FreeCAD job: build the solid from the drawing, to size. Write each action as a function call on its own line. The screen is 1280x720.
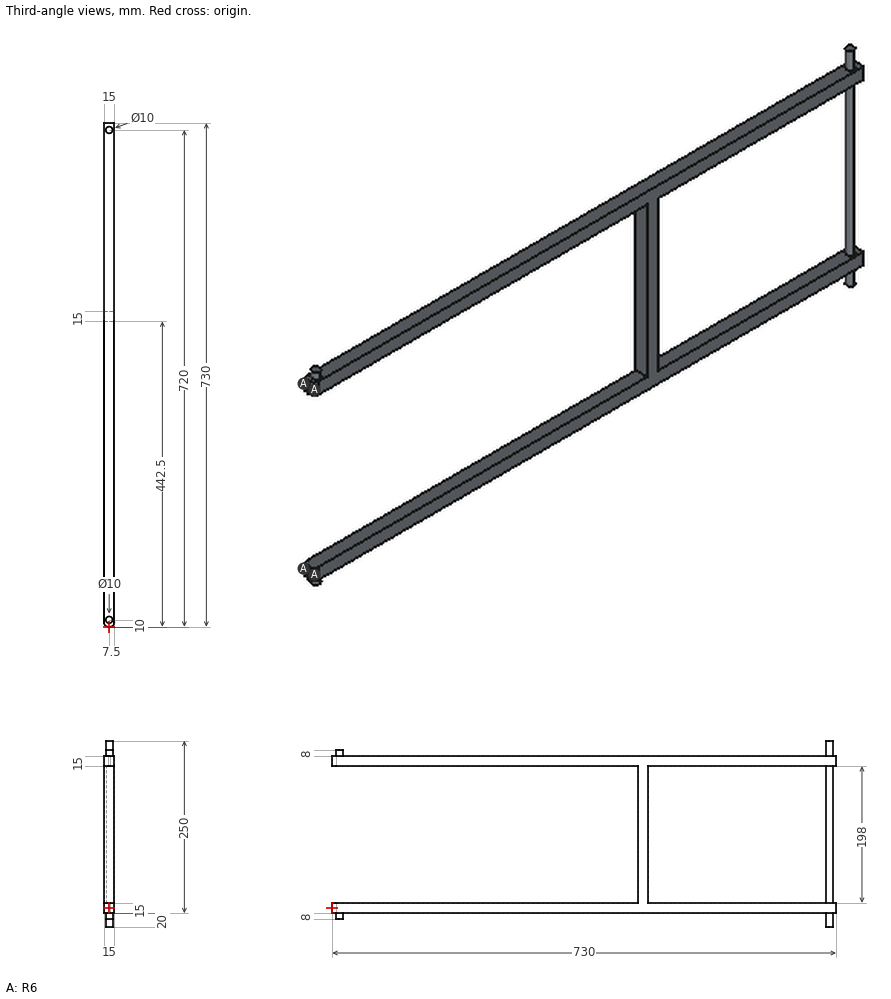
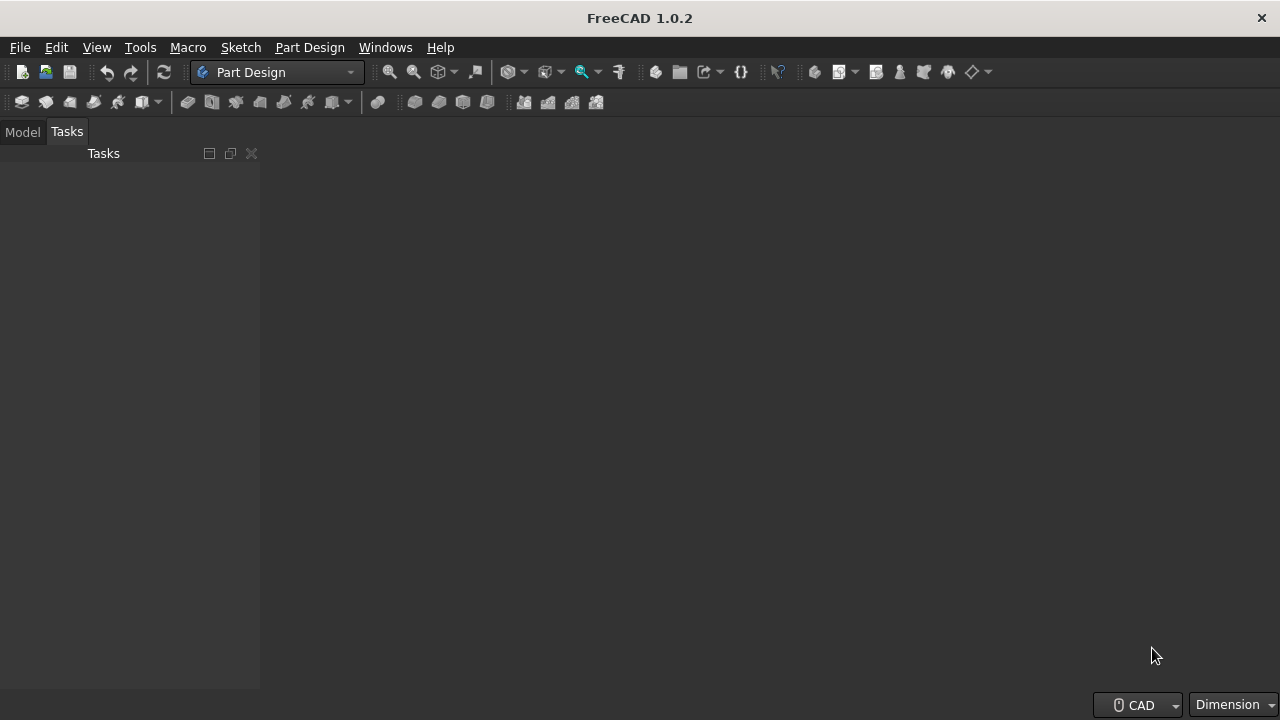
key(ctrl+n)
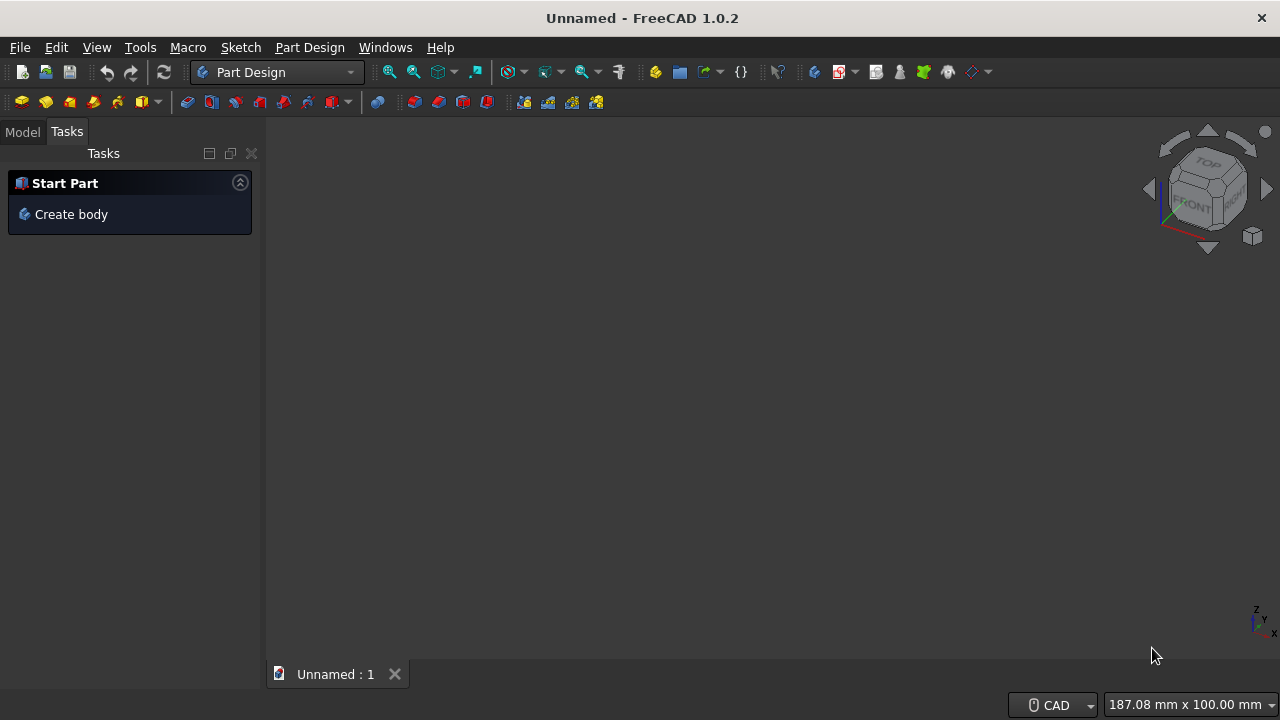
click(840, 72)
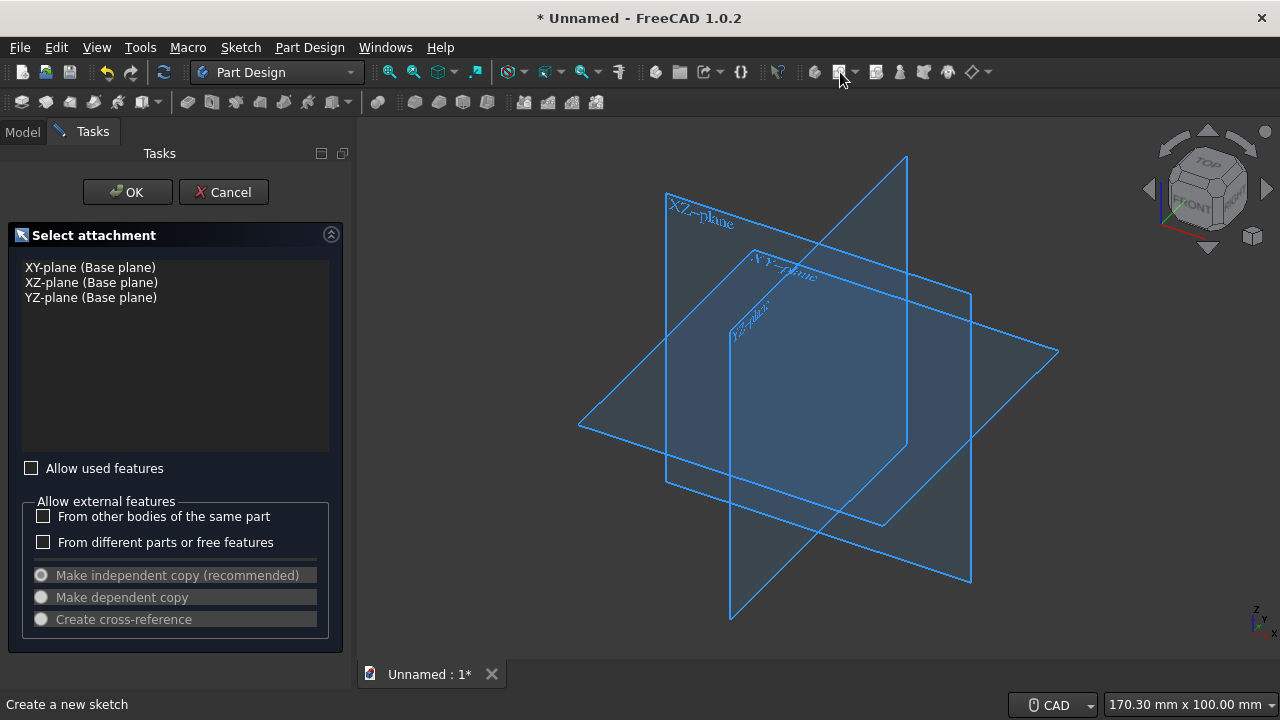
click(82, 282)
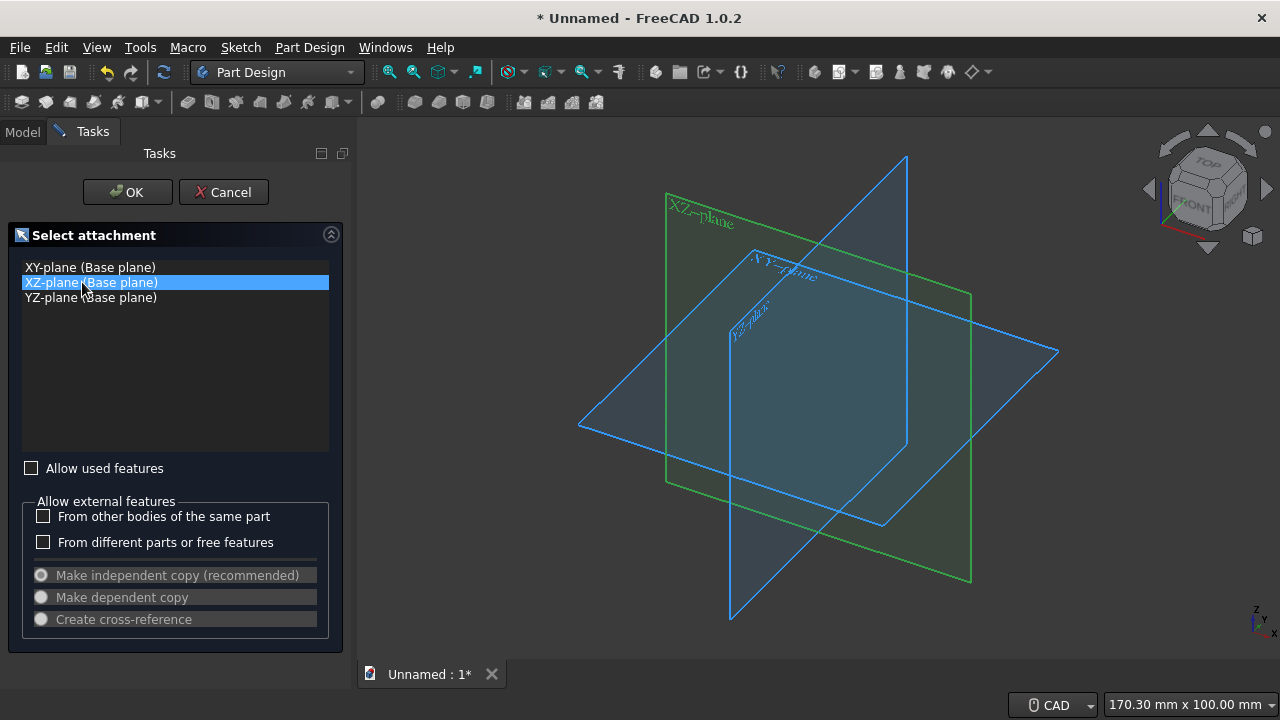
click(128, 192)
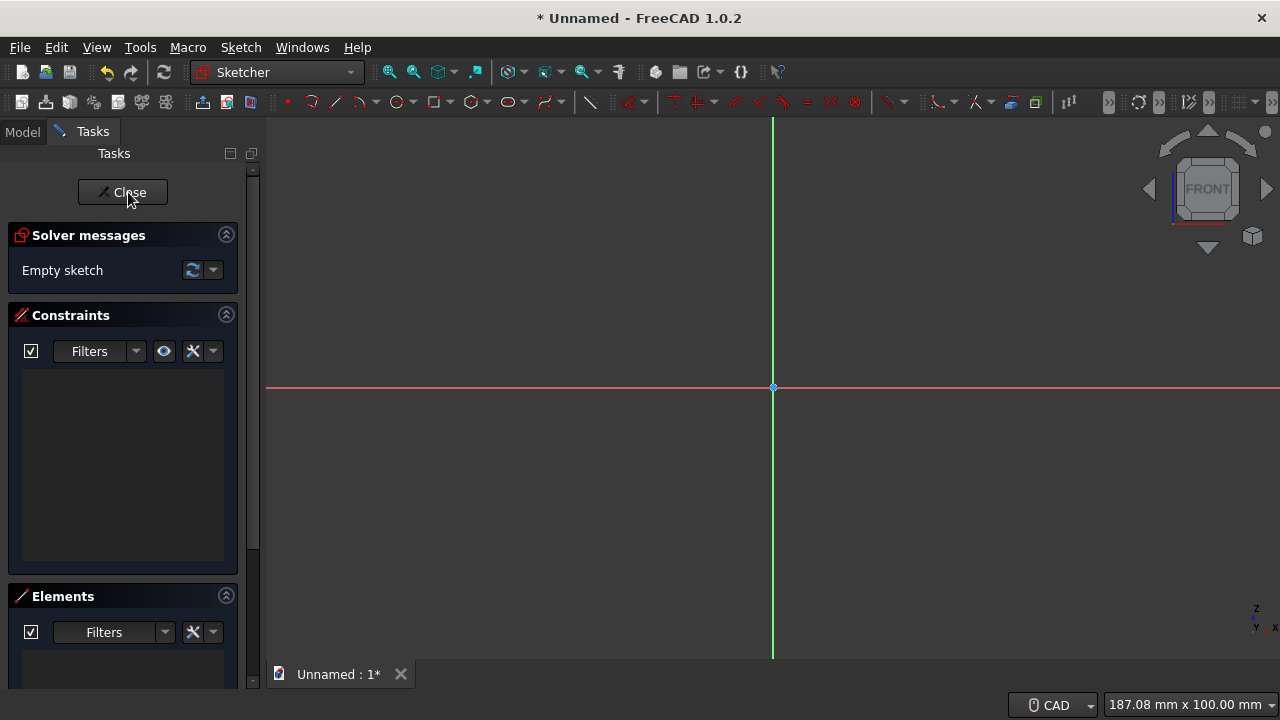
scroll(795, 388, up, 7)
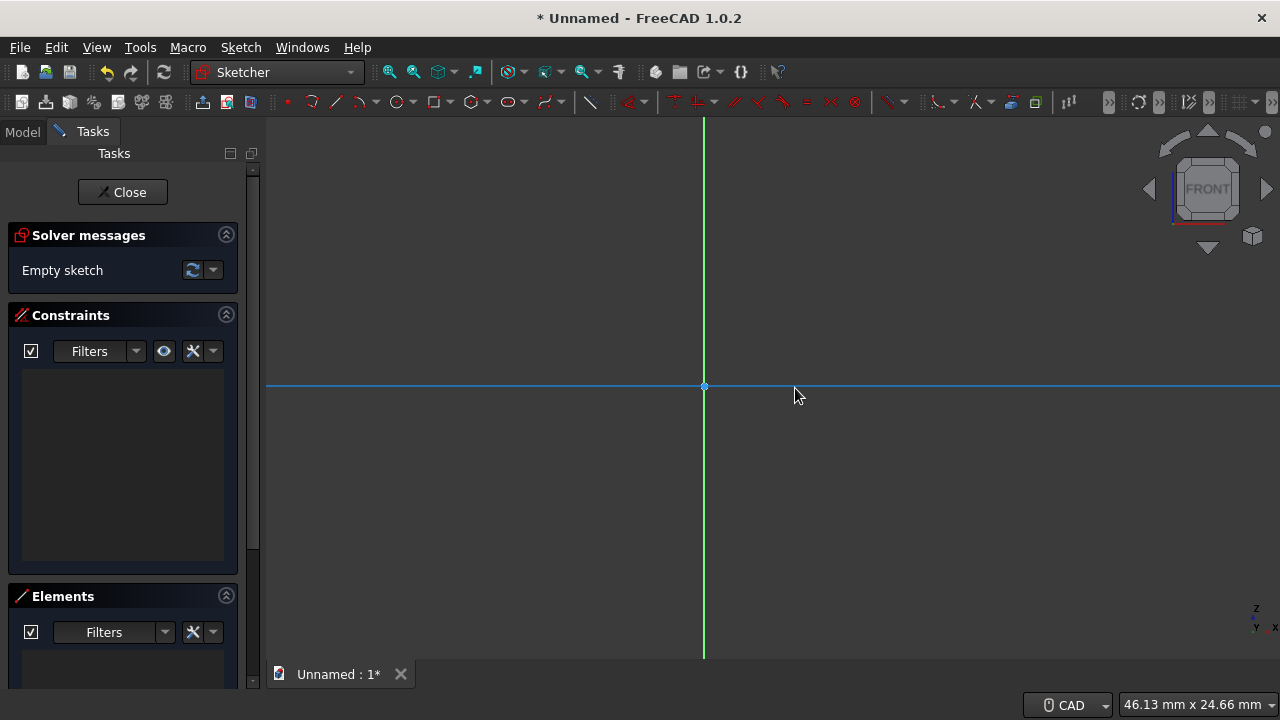
click(452, 102)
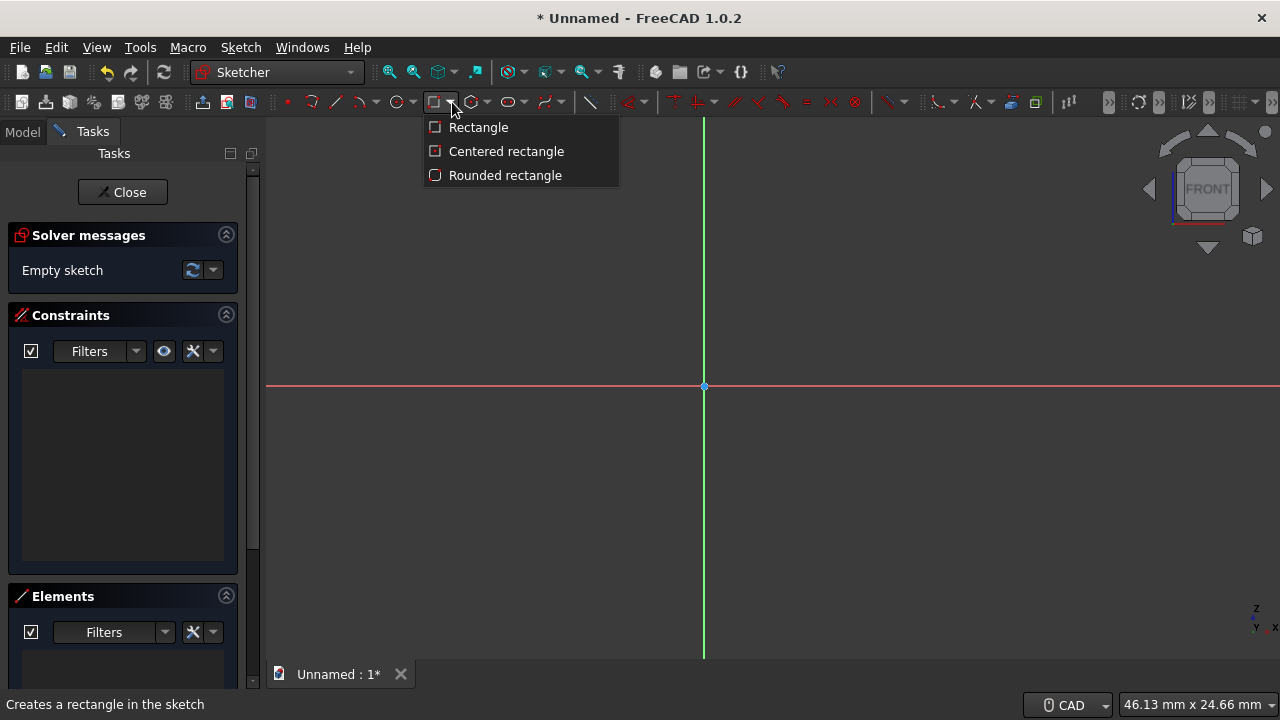
click(522, 151)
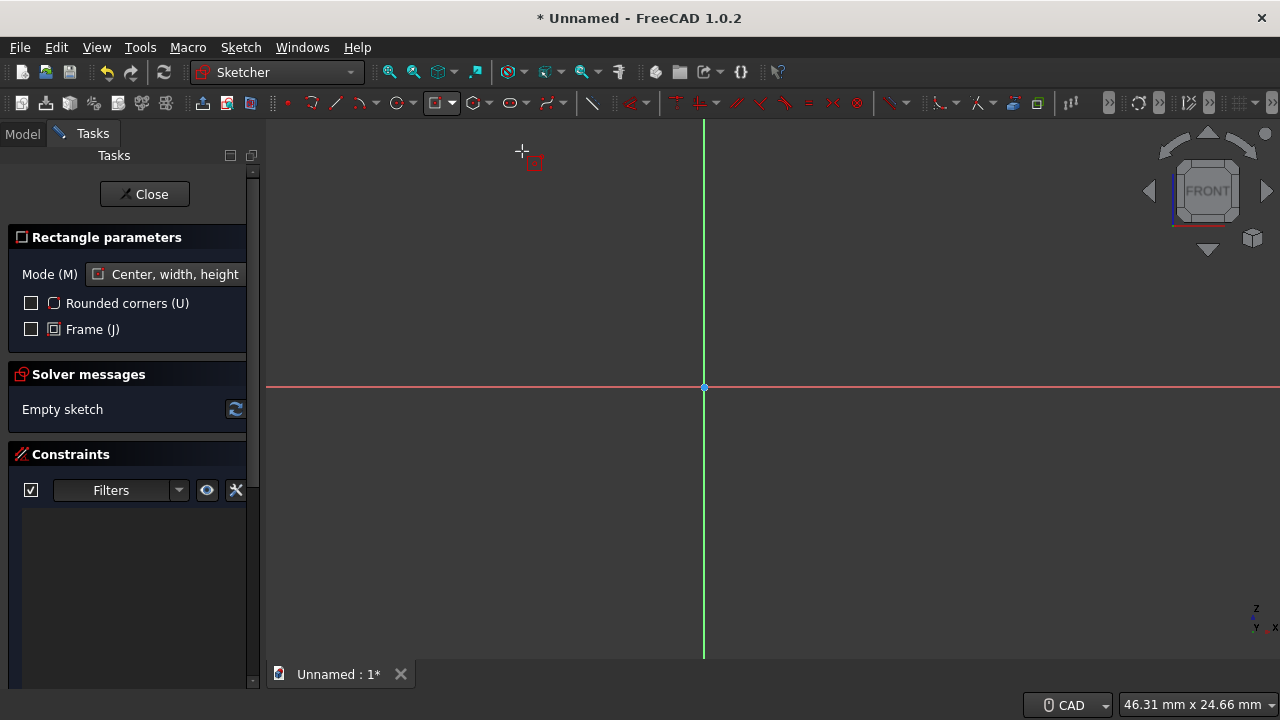
click(704, 387)
move(869, 223)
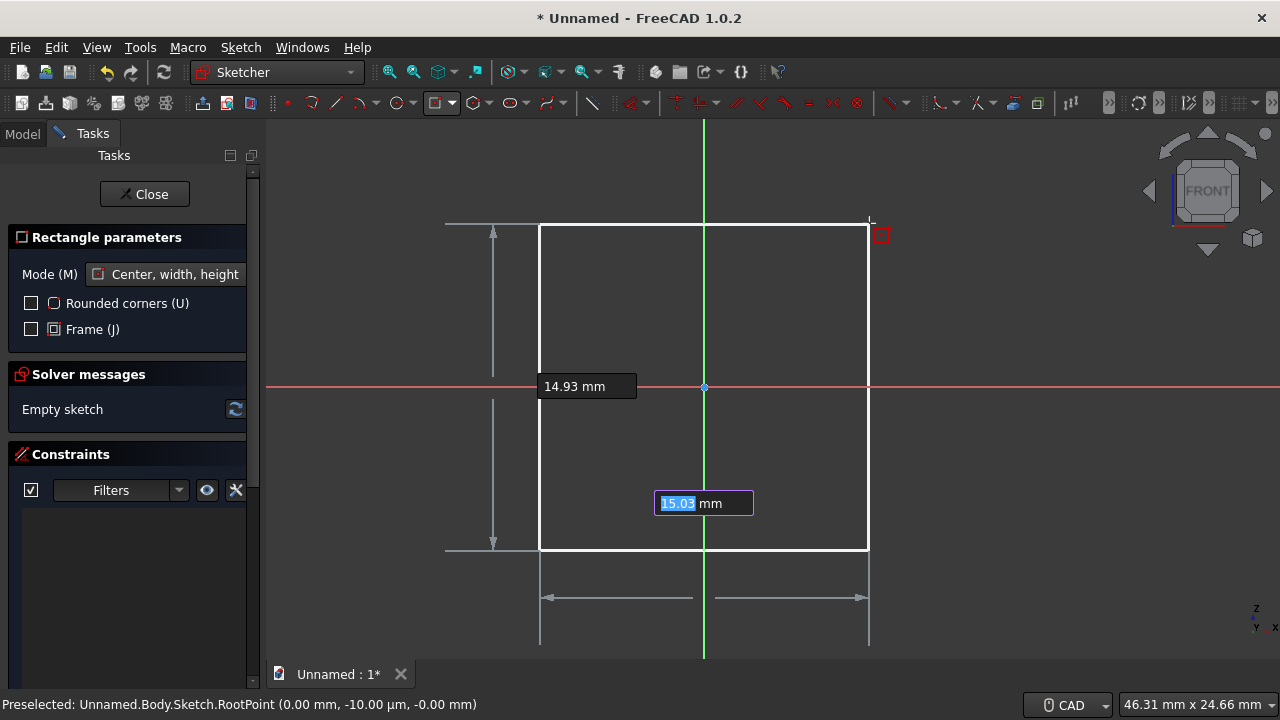
text(15)
key(Tab)
text(15)
key(Return)
key(Escape)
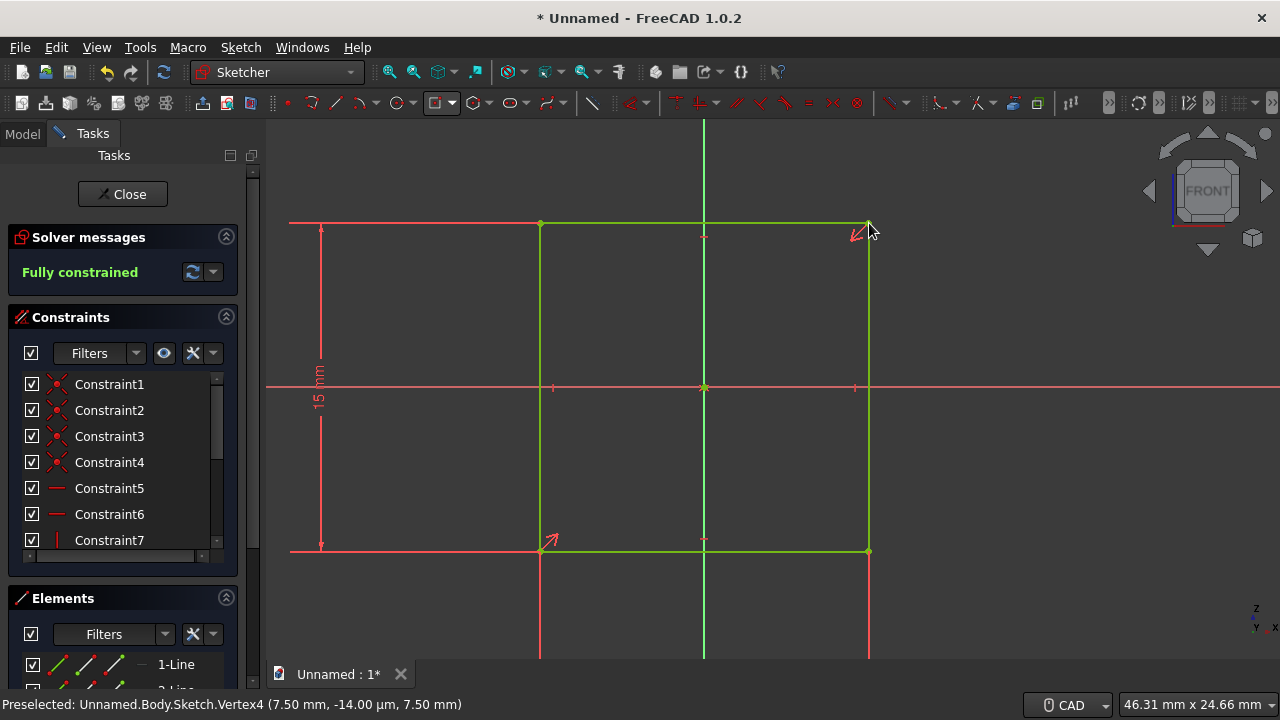
click(123, 194)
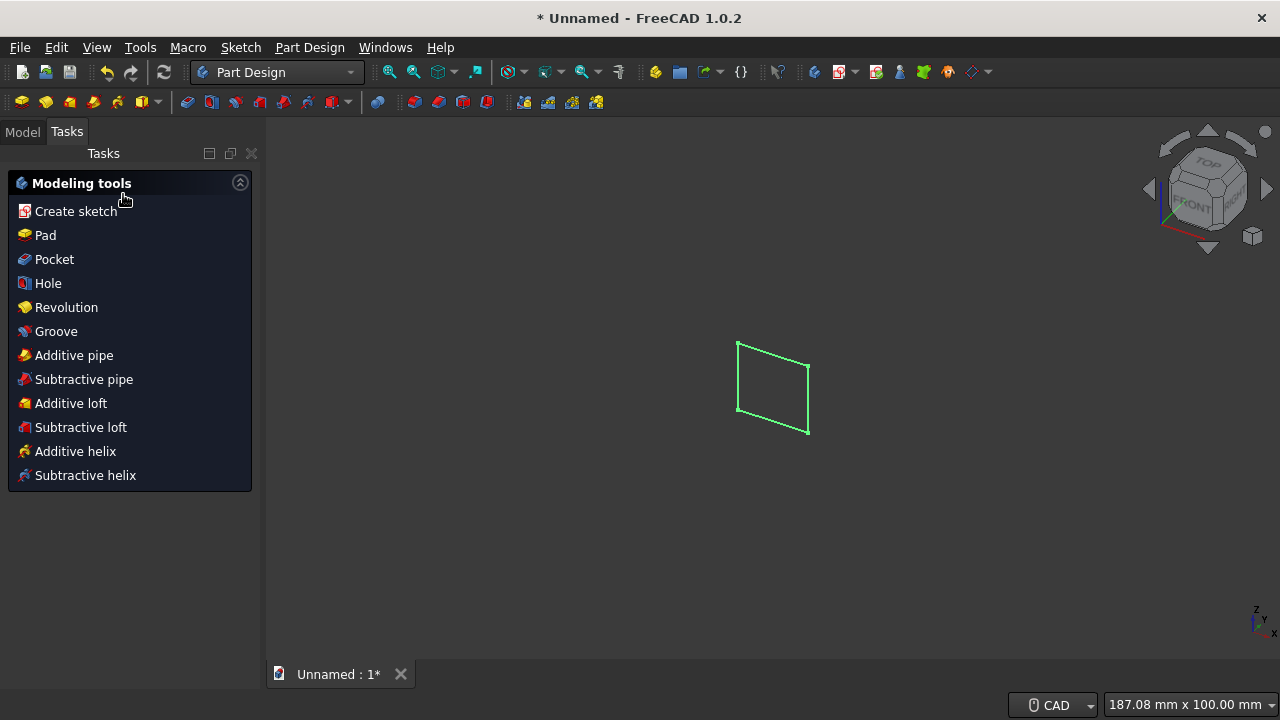
click(22, 102)